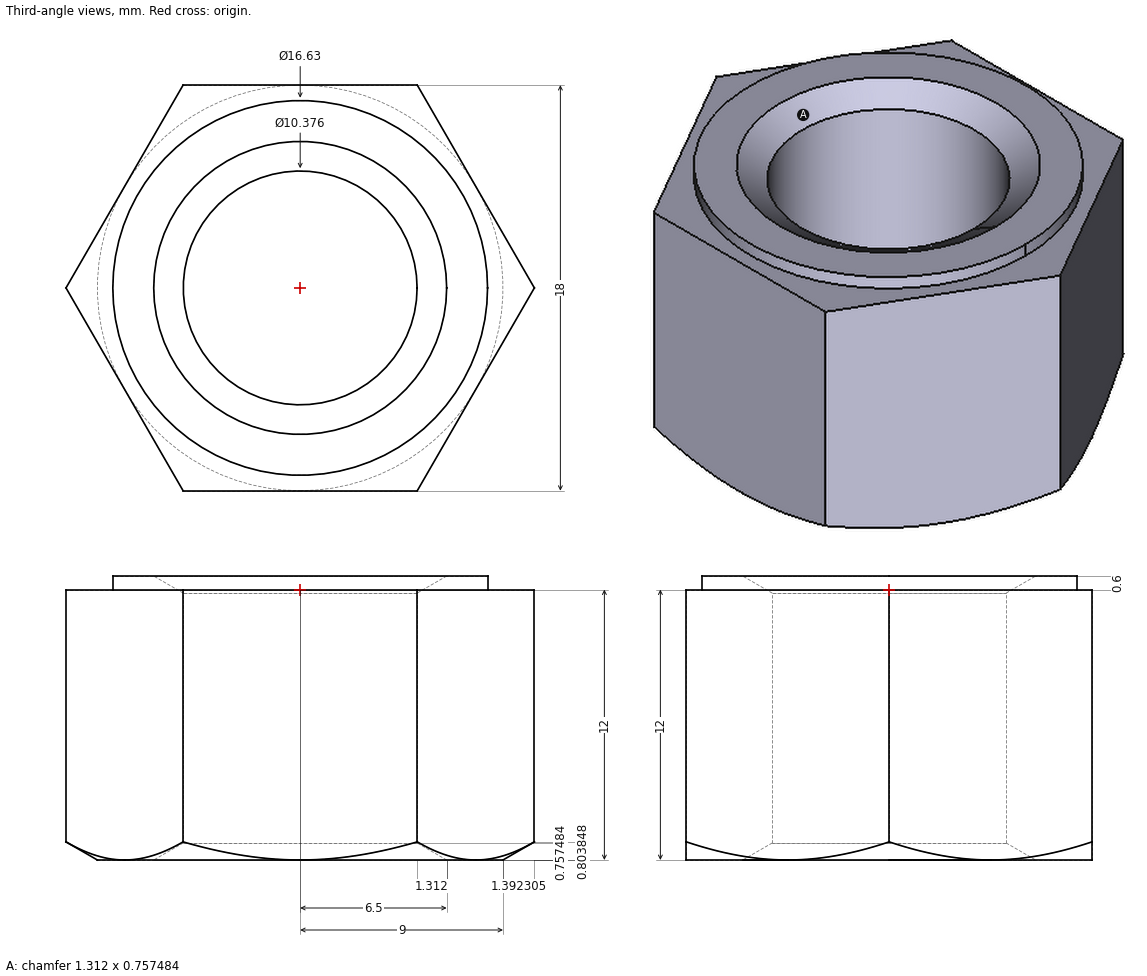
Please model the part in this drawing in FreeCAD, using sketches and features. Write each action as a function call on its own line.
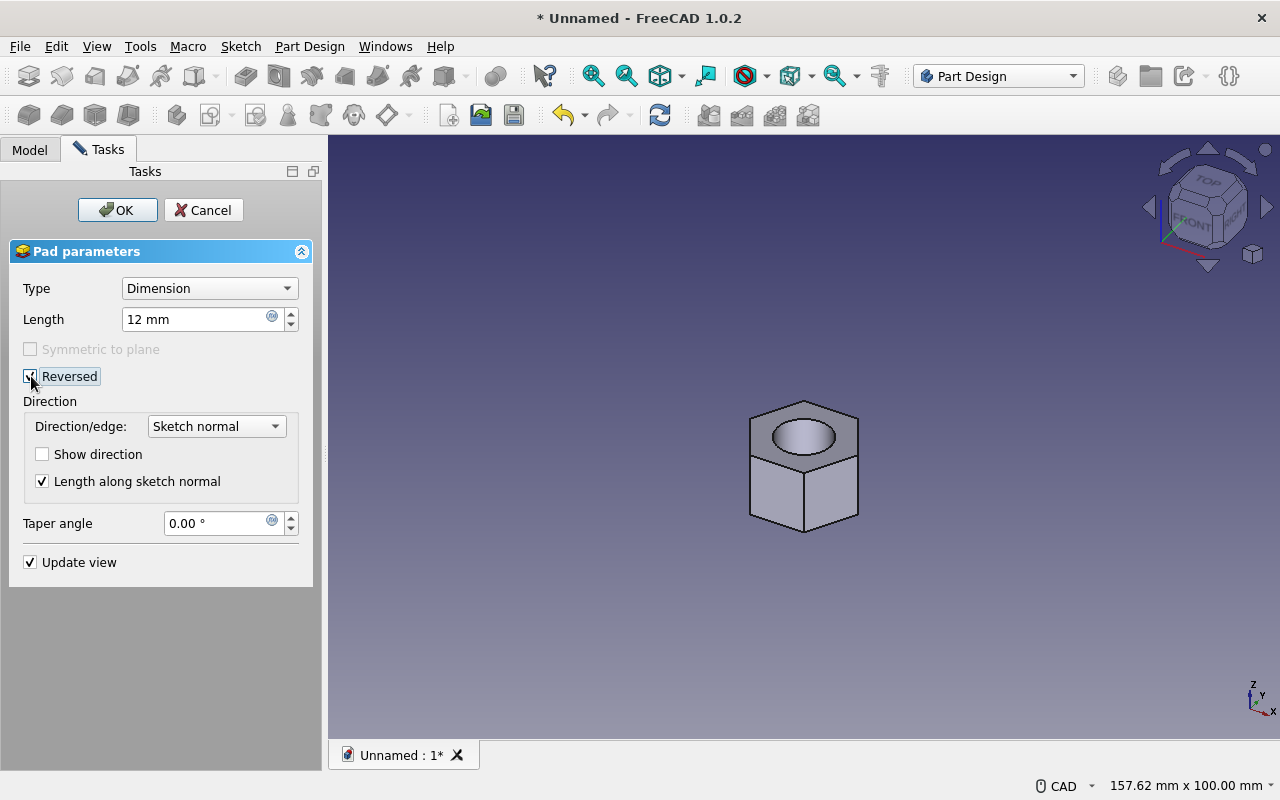
click(118, 210)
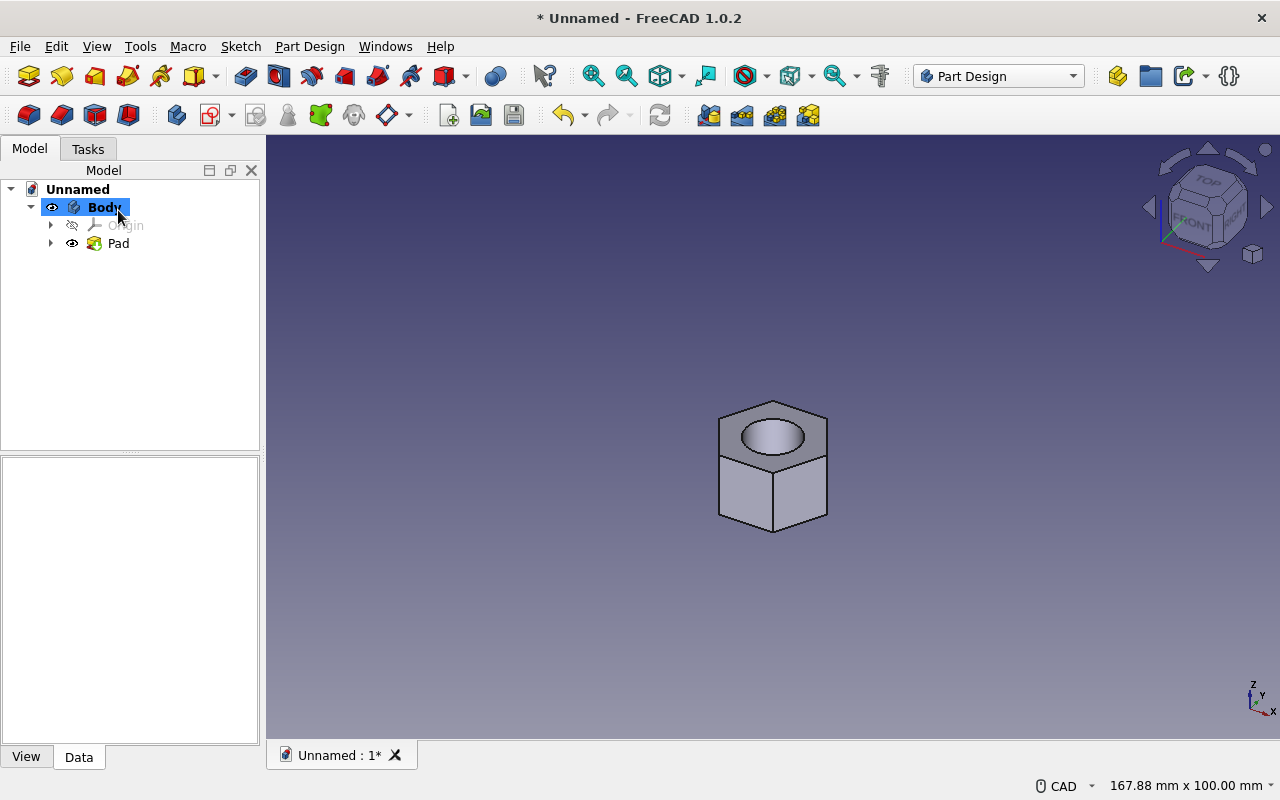
click(594, 76)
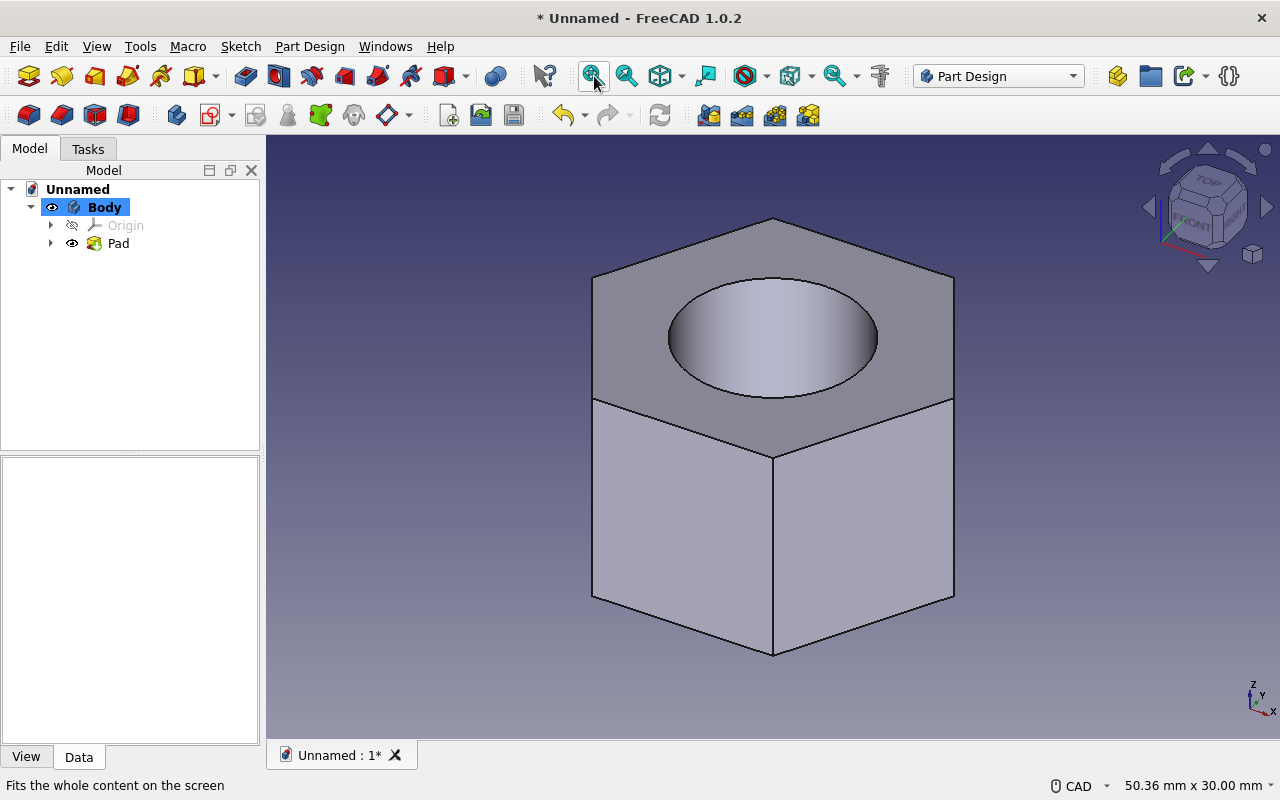
click(210, 116)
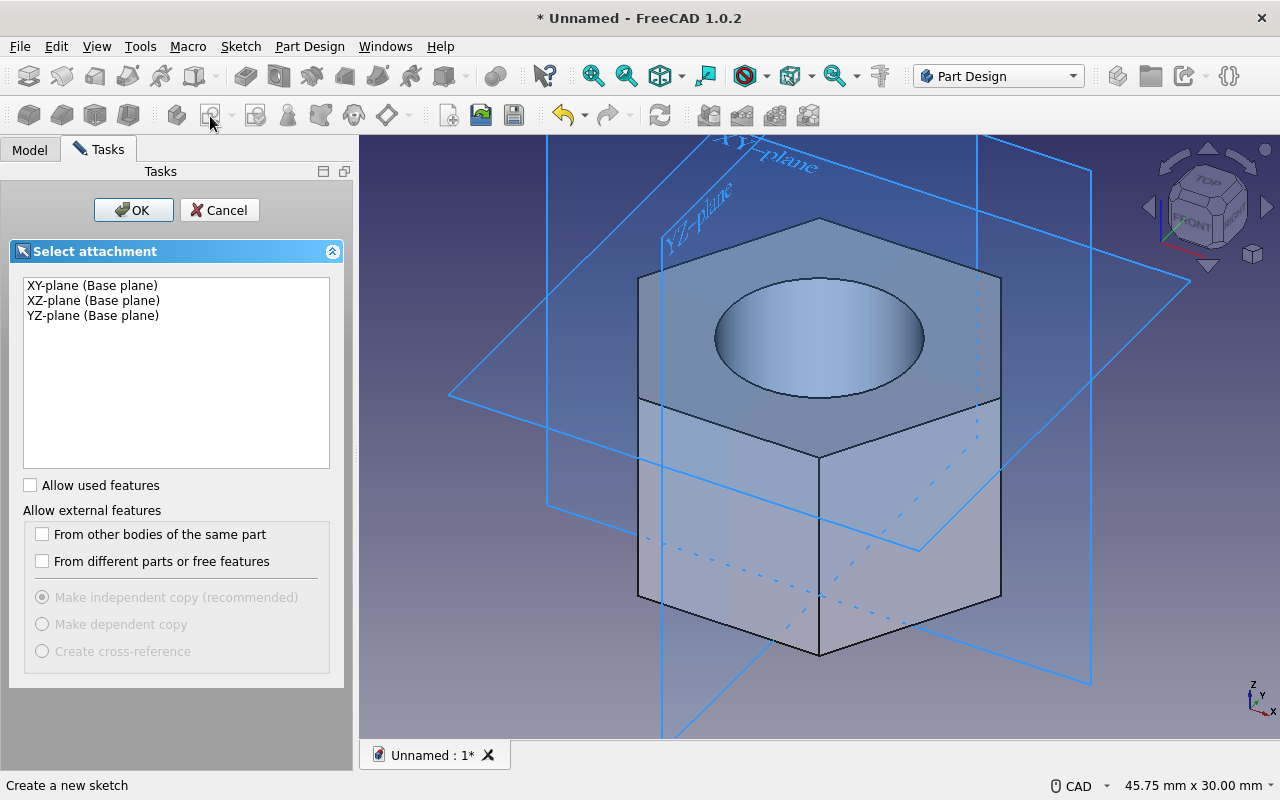
click(84, 300)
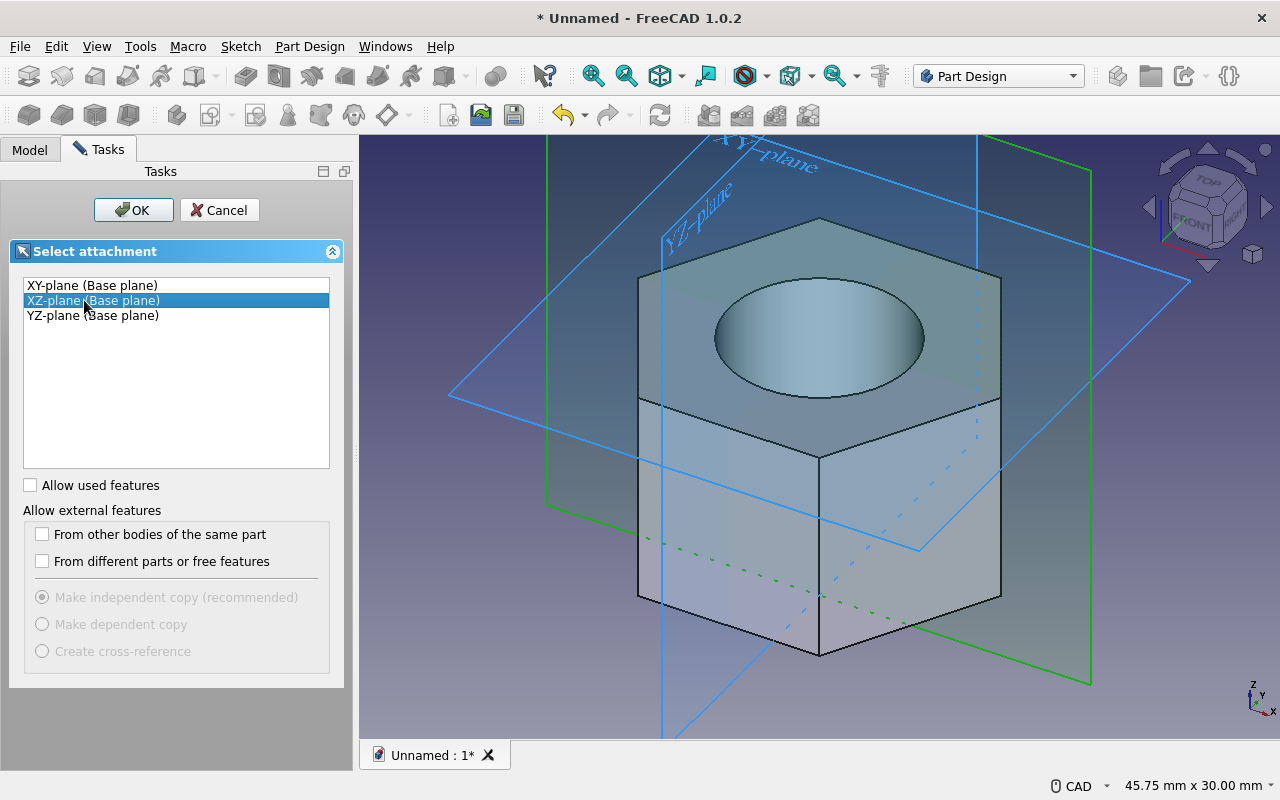
click(134, 210)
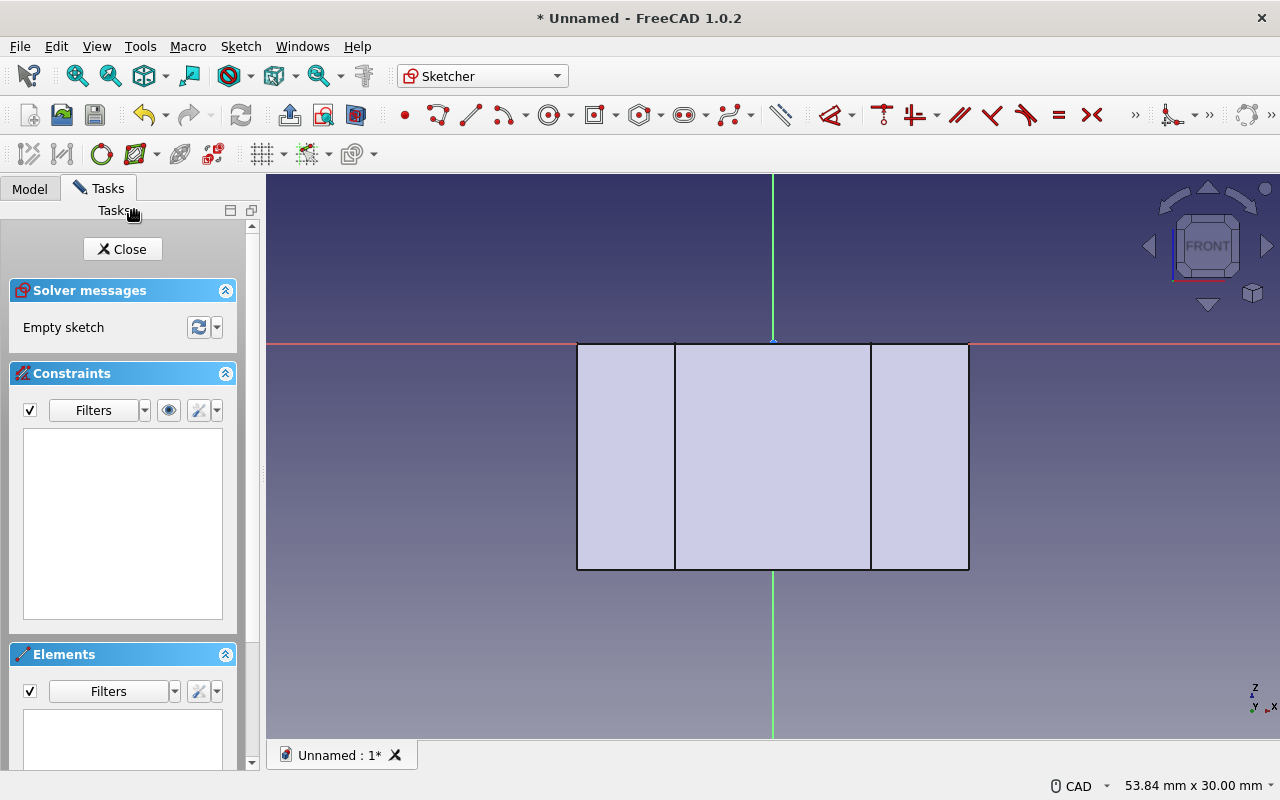
key(q)
key(s)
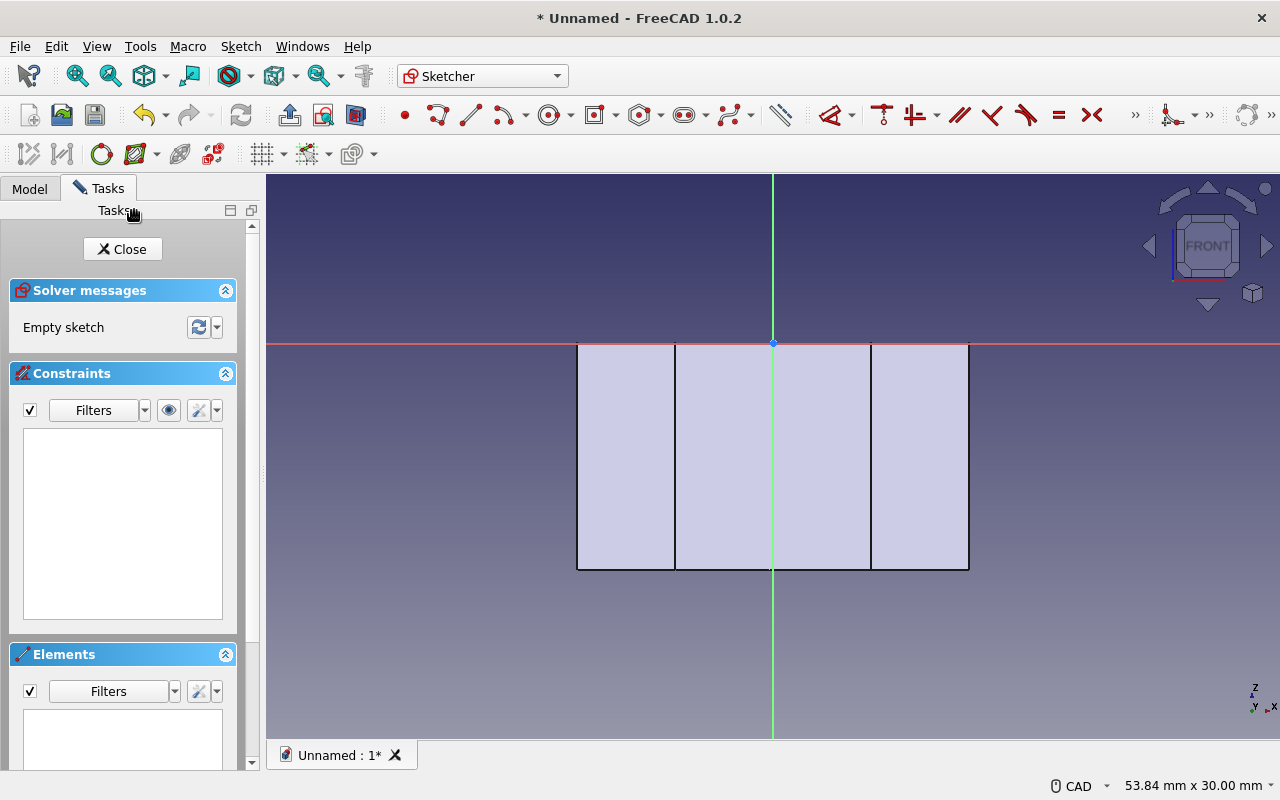
scroll(969, 567, up, 15)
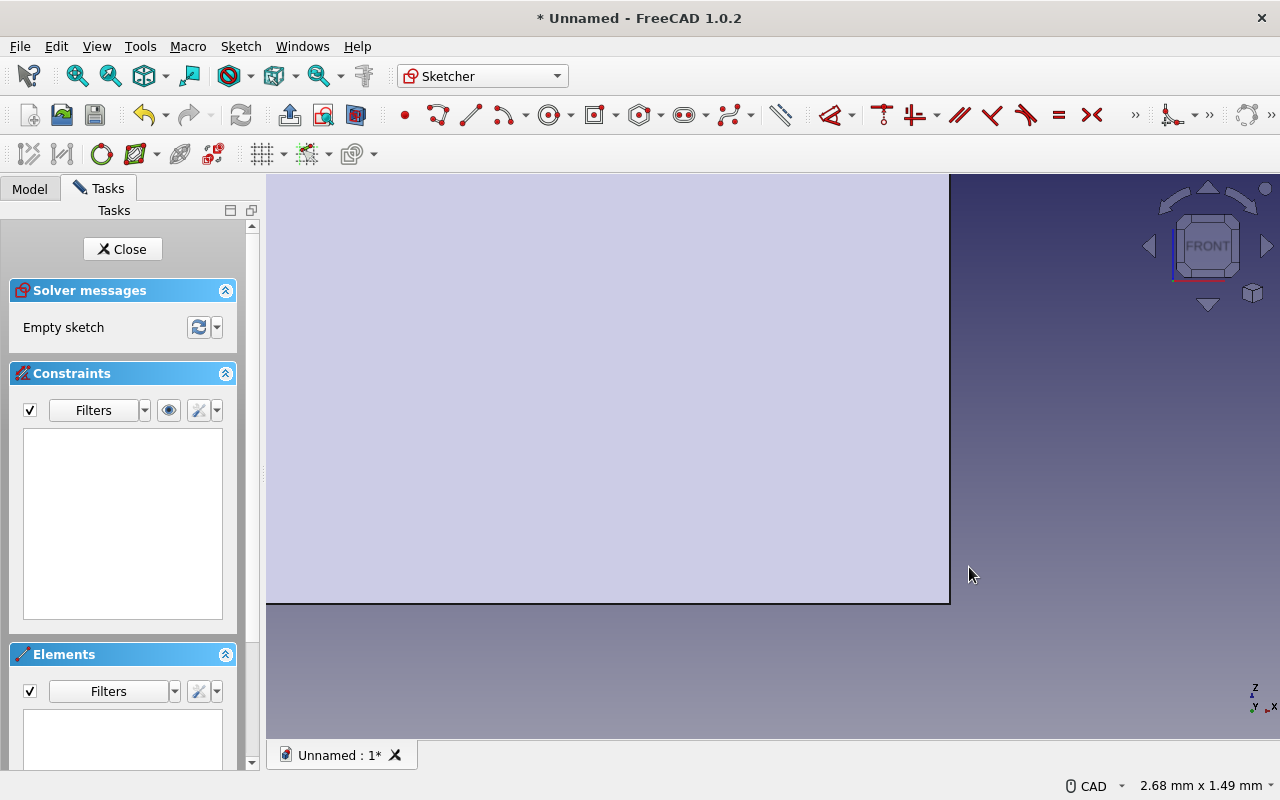
key(g)
key(m)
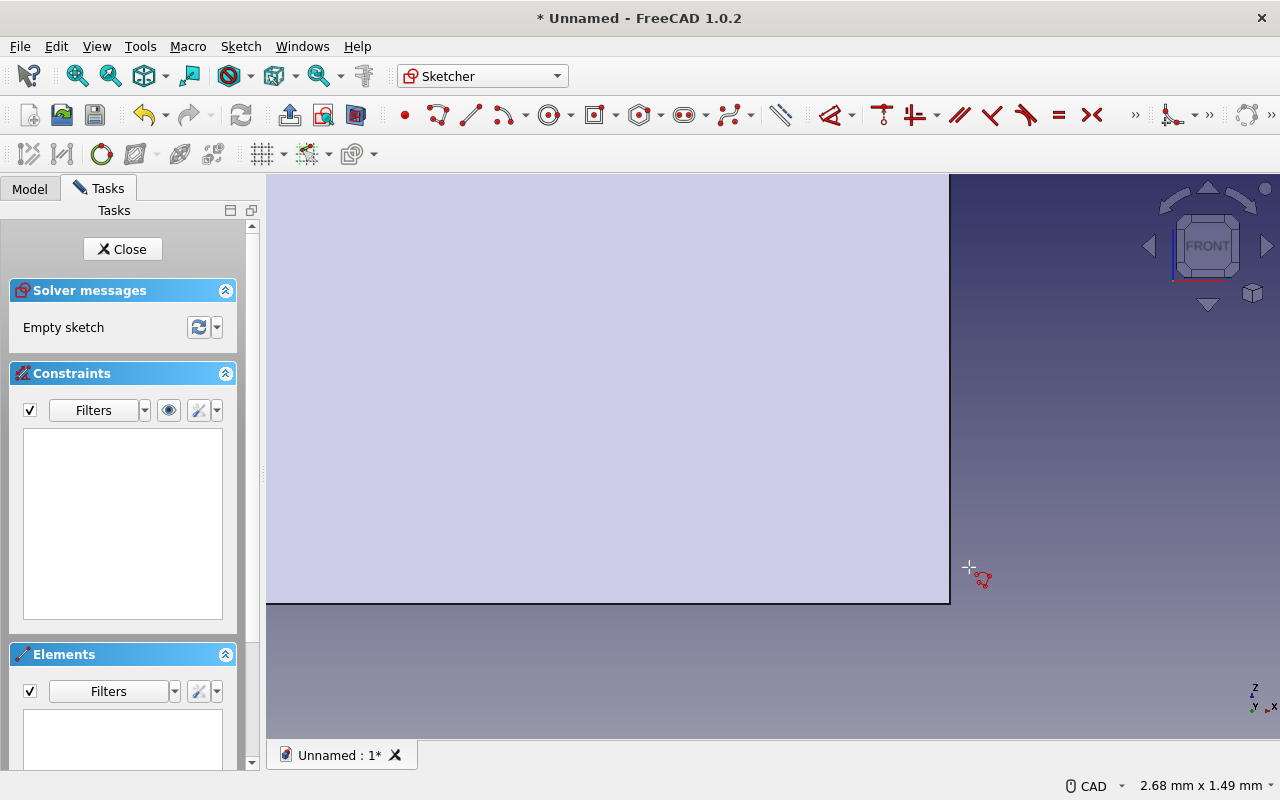
click(423, 604)
click(950, 300)
click(950, 604)
click(423, 605)
key(Escape)
key(Escape)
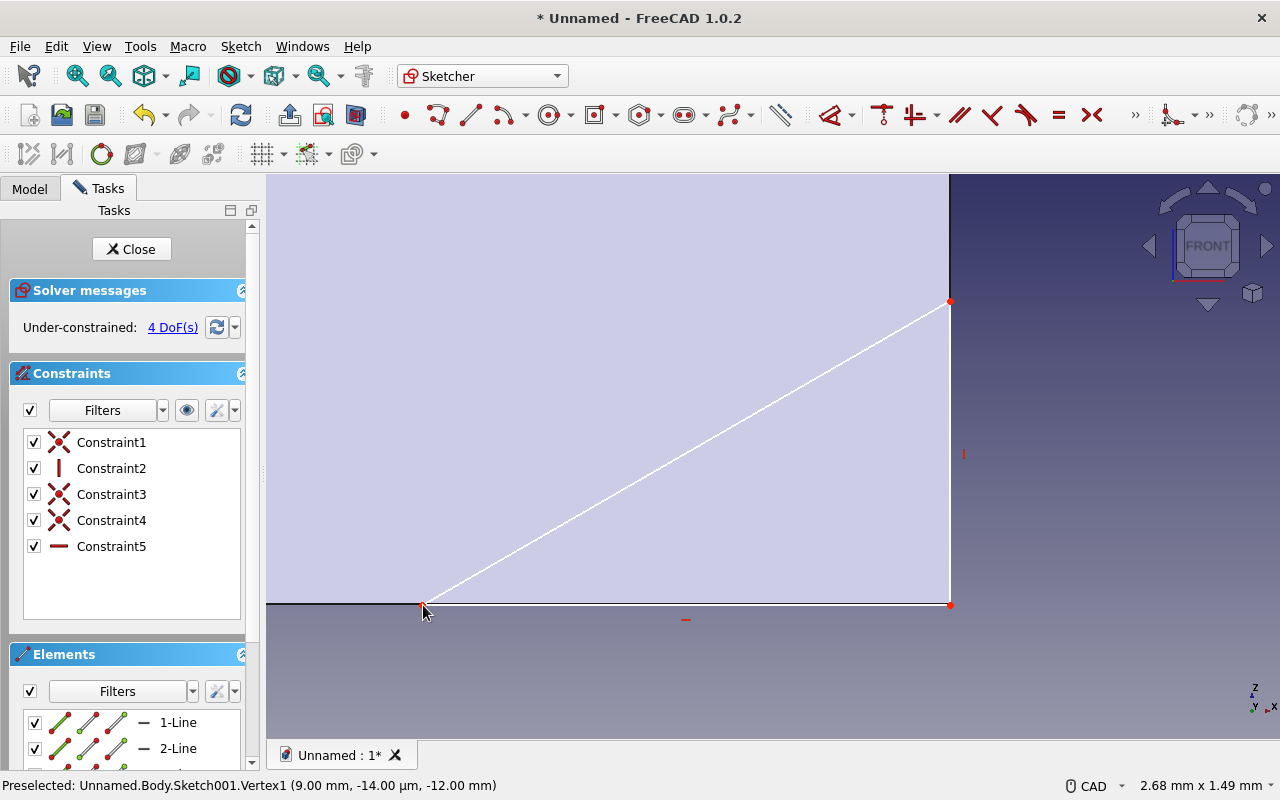
key(d)